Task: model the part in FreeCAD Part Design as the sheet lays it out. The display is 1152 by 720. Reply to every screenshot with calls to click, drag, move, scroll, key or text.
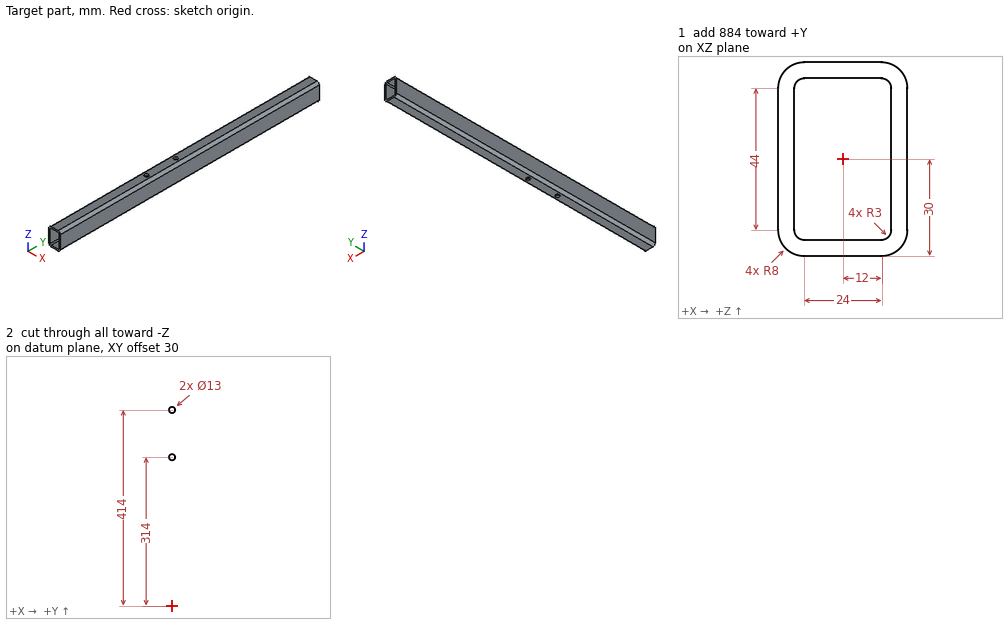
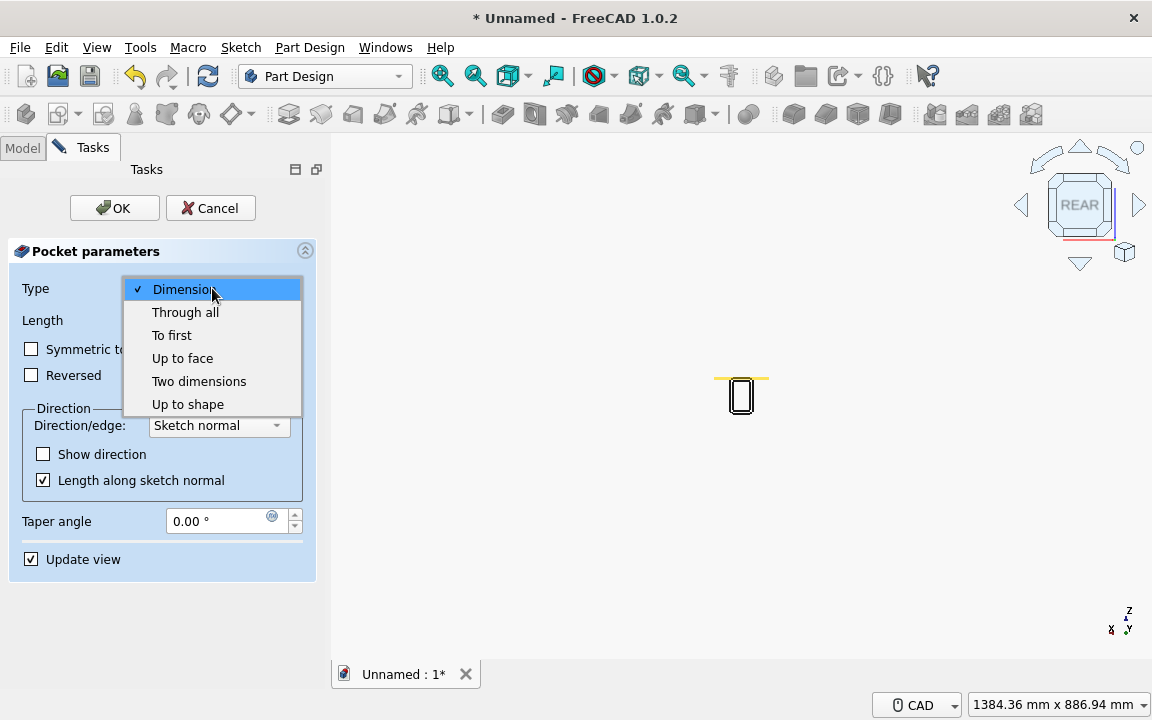
click(212, 312)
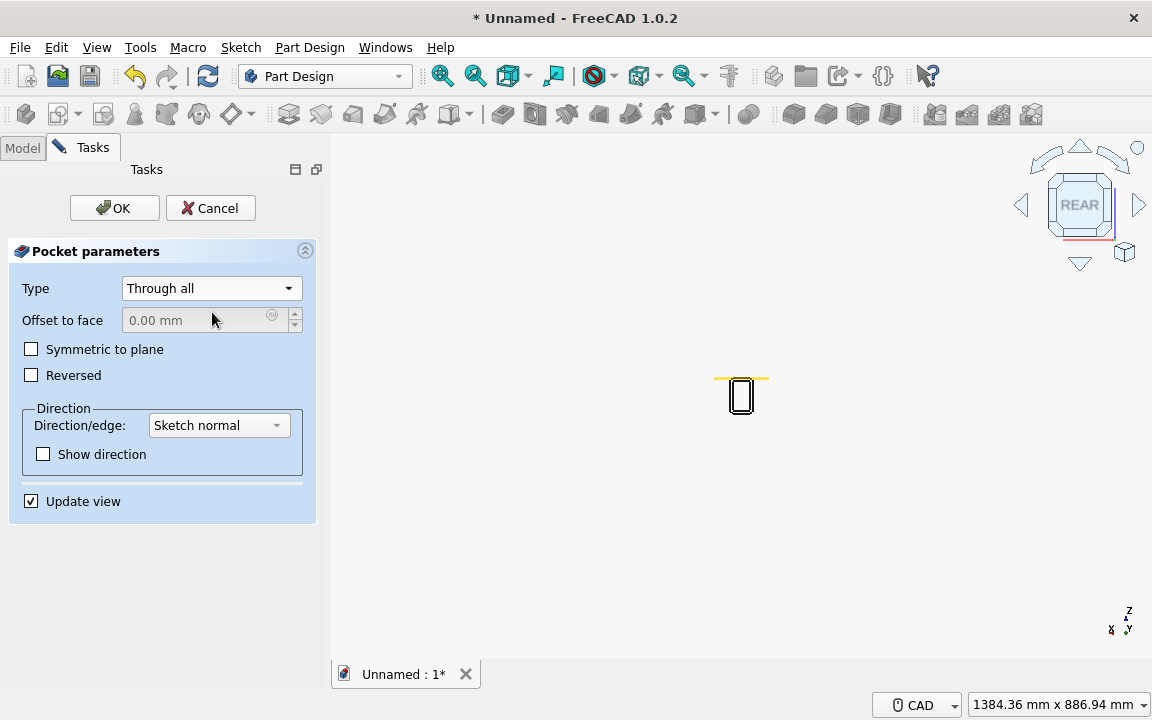
click(115, 208)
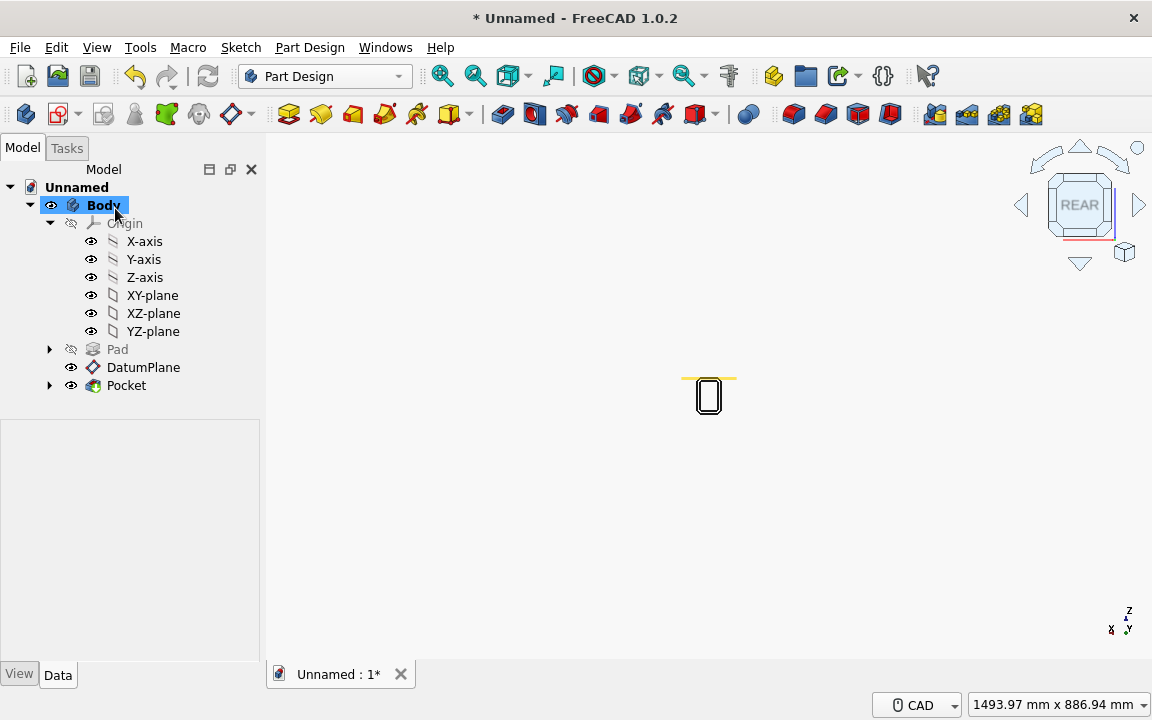
click(116, 367)
key(space)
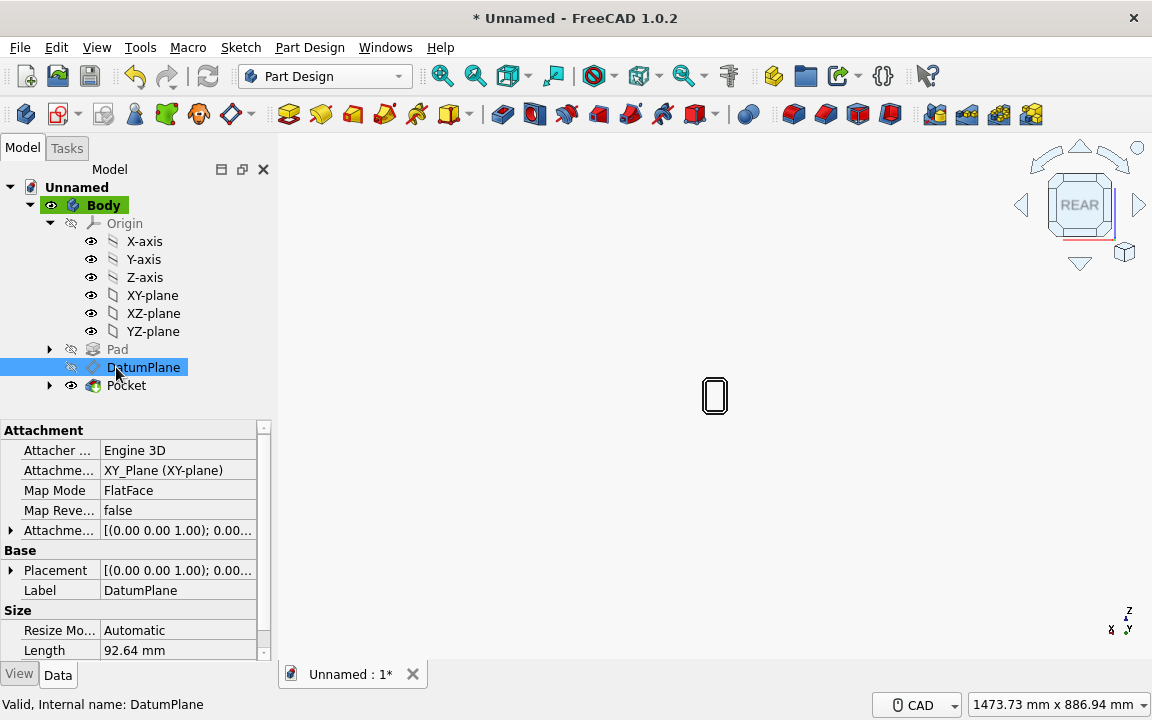
key(0)